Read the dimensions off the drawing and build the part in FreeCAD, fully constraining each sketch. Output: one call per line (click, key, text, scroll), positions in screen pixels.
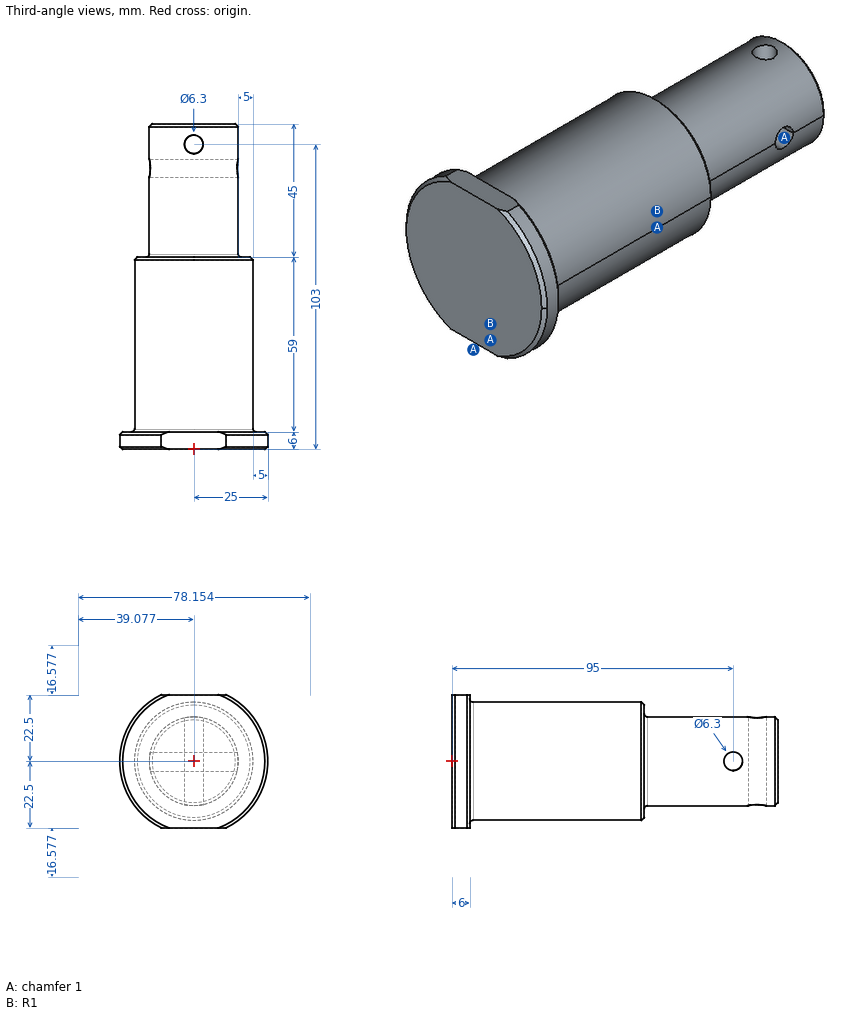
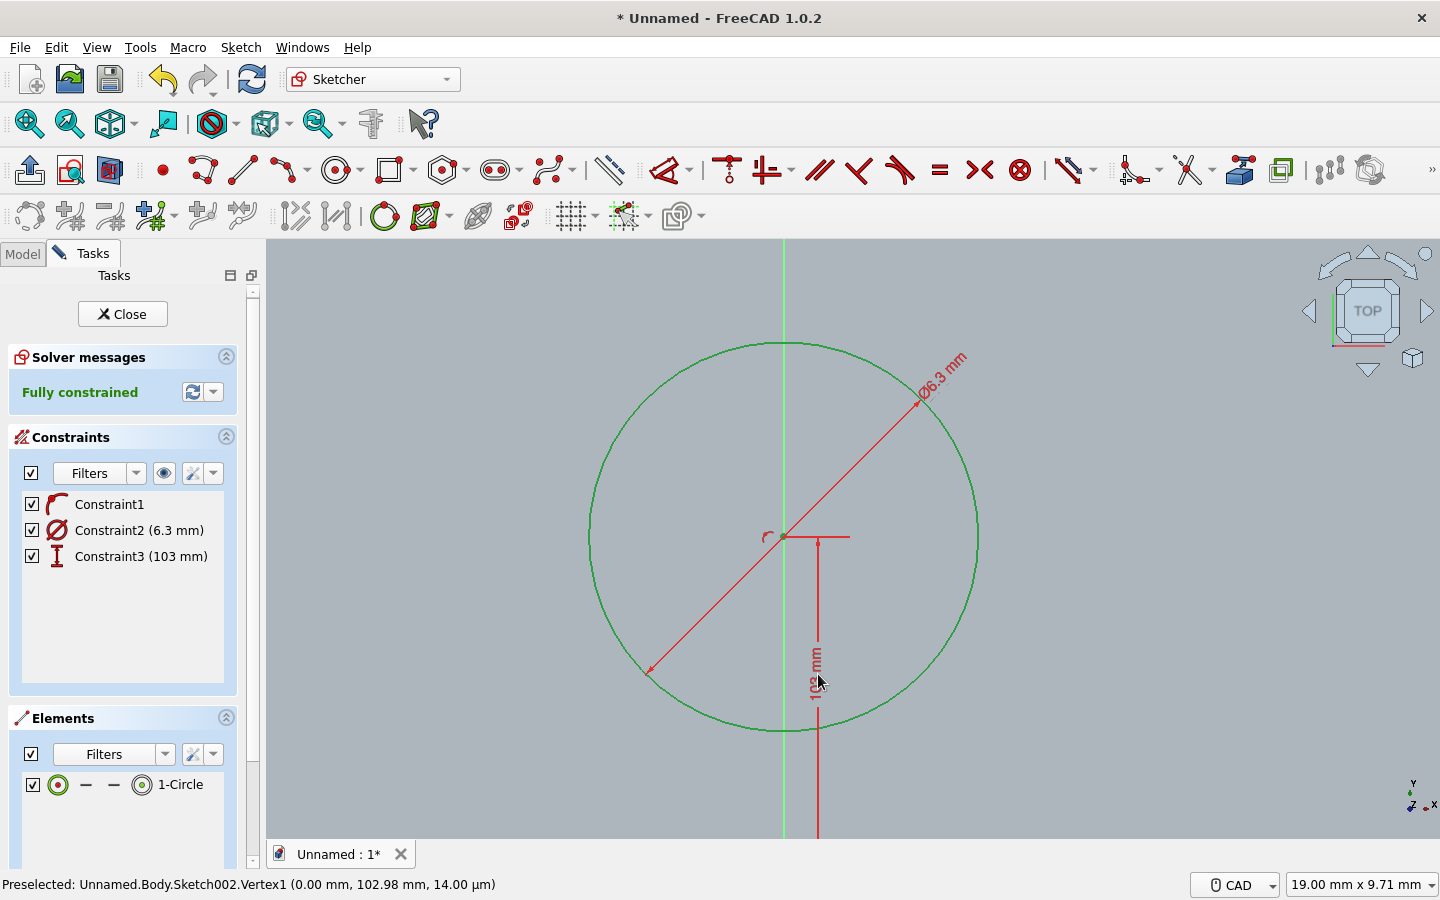
click(123, 314)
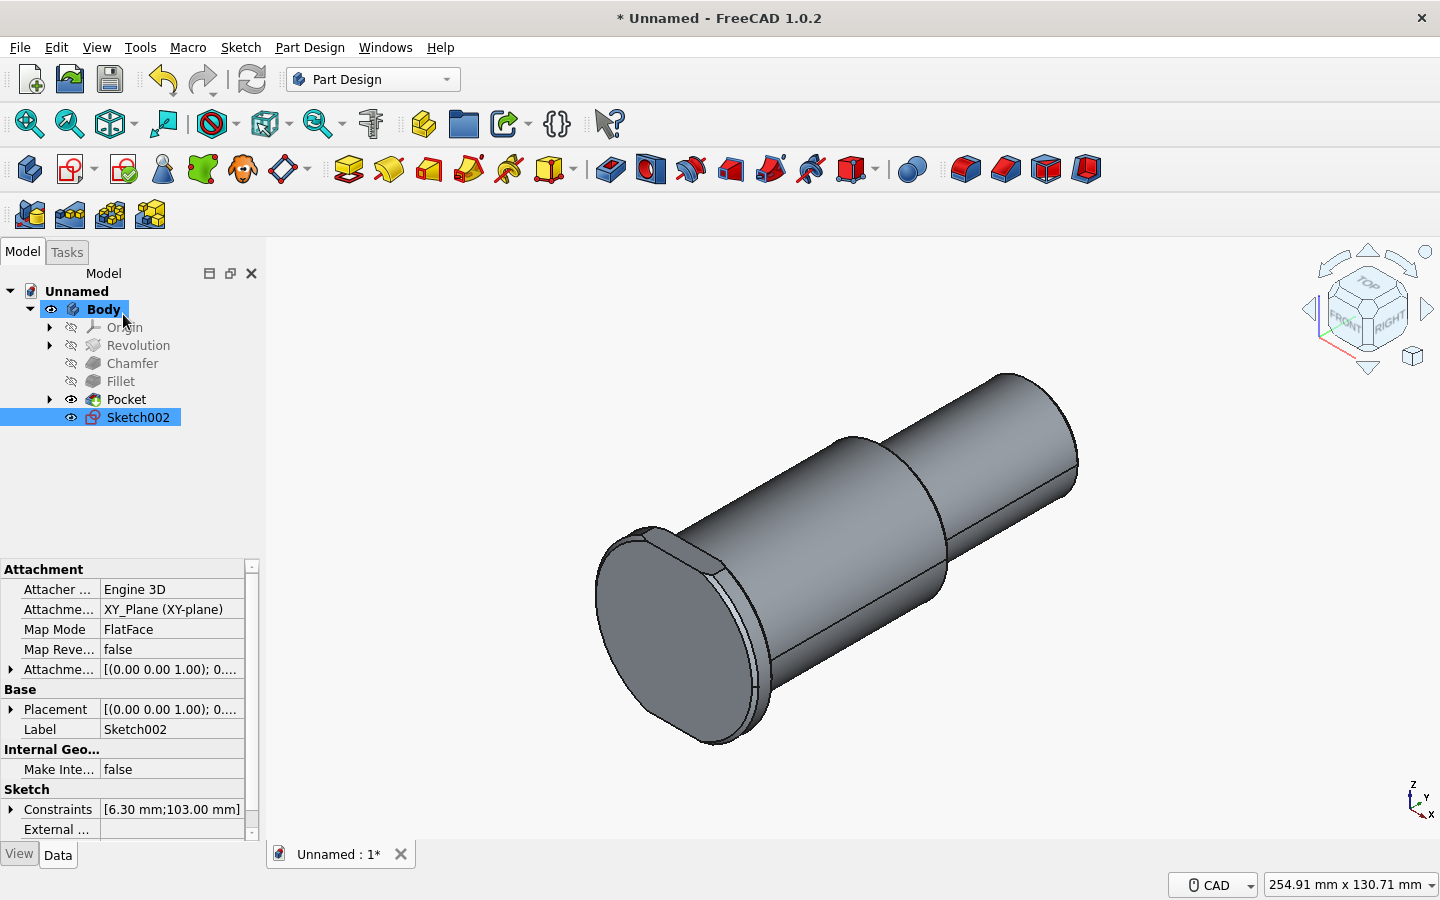
click(612, 170)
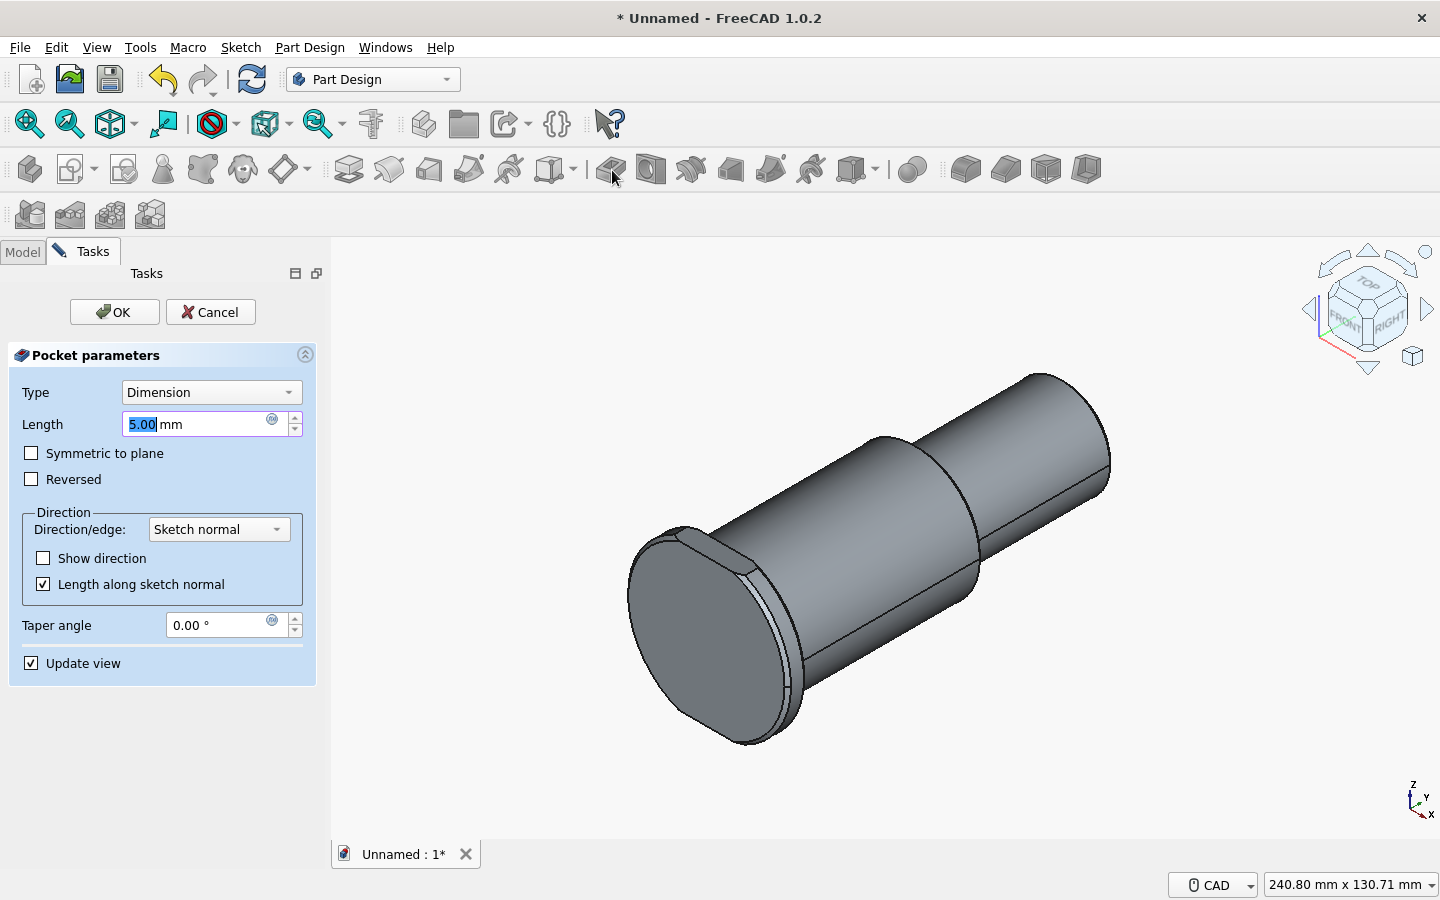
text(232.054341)
key(Tab)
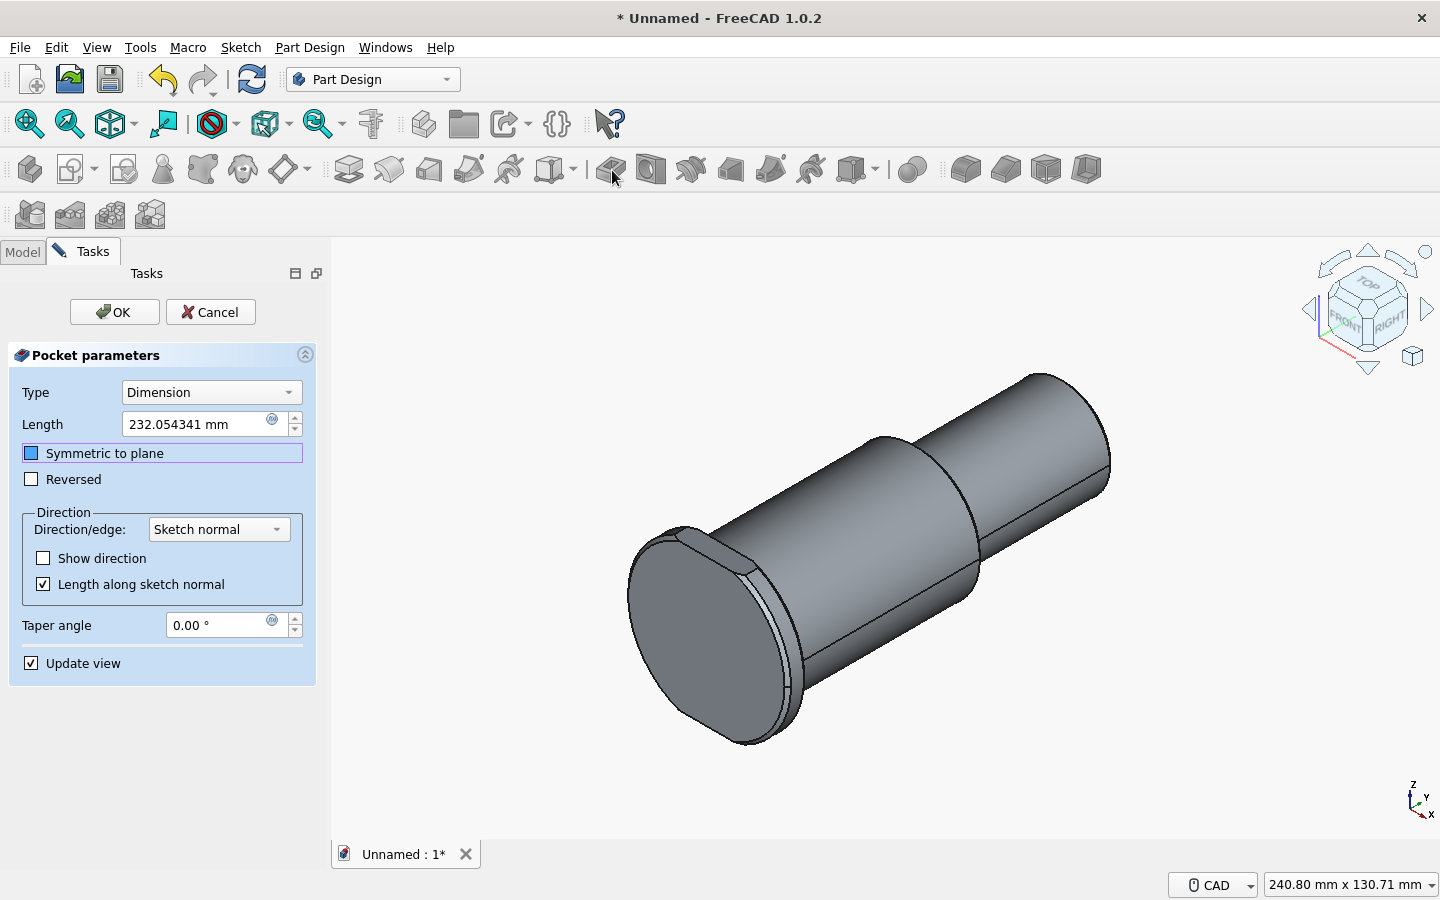
click(30, 453)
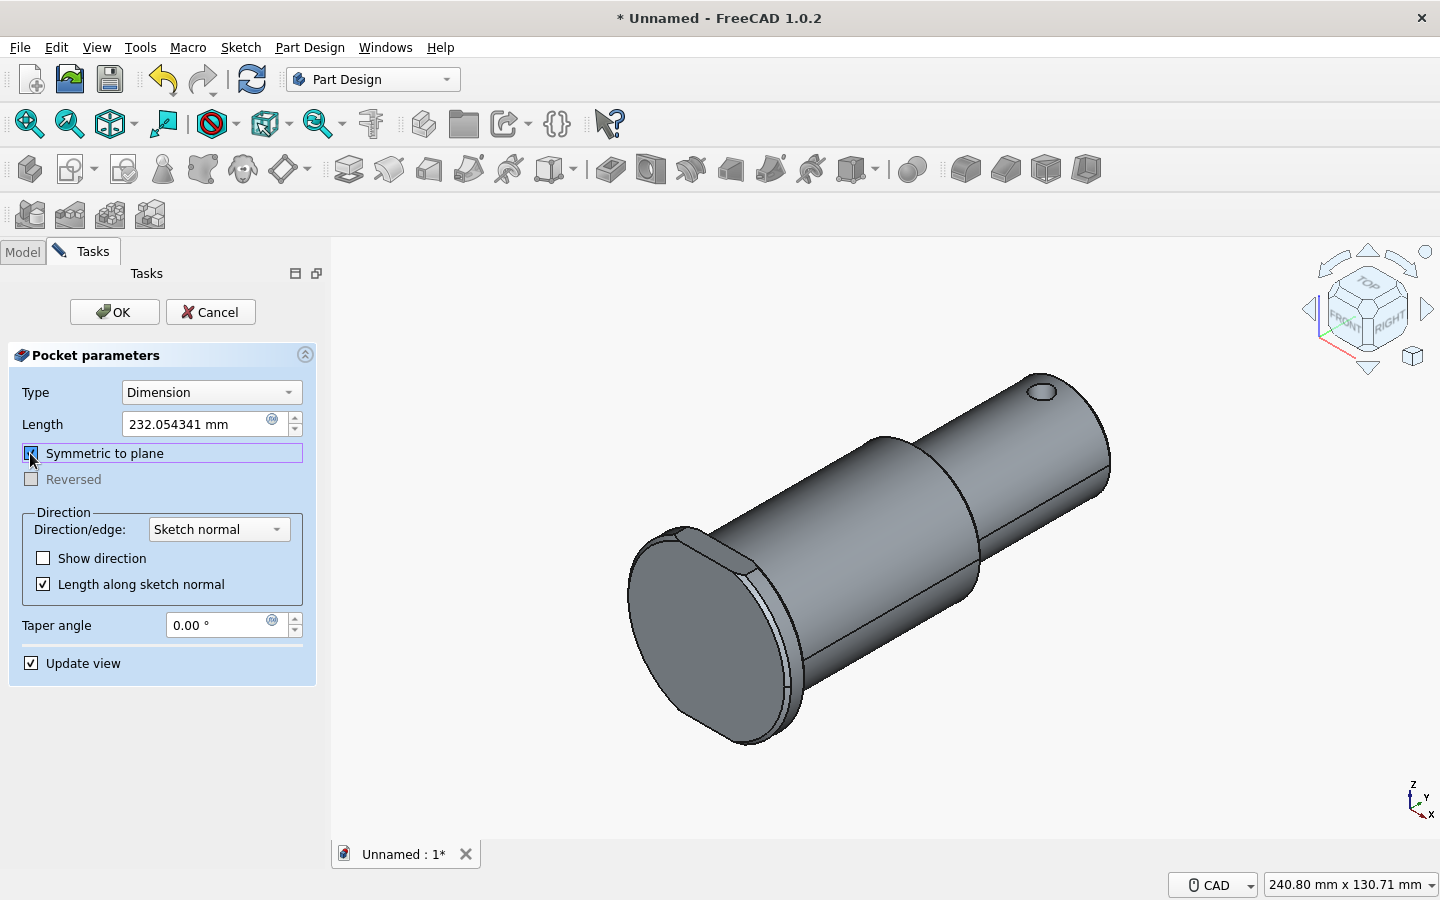
click(115, 312)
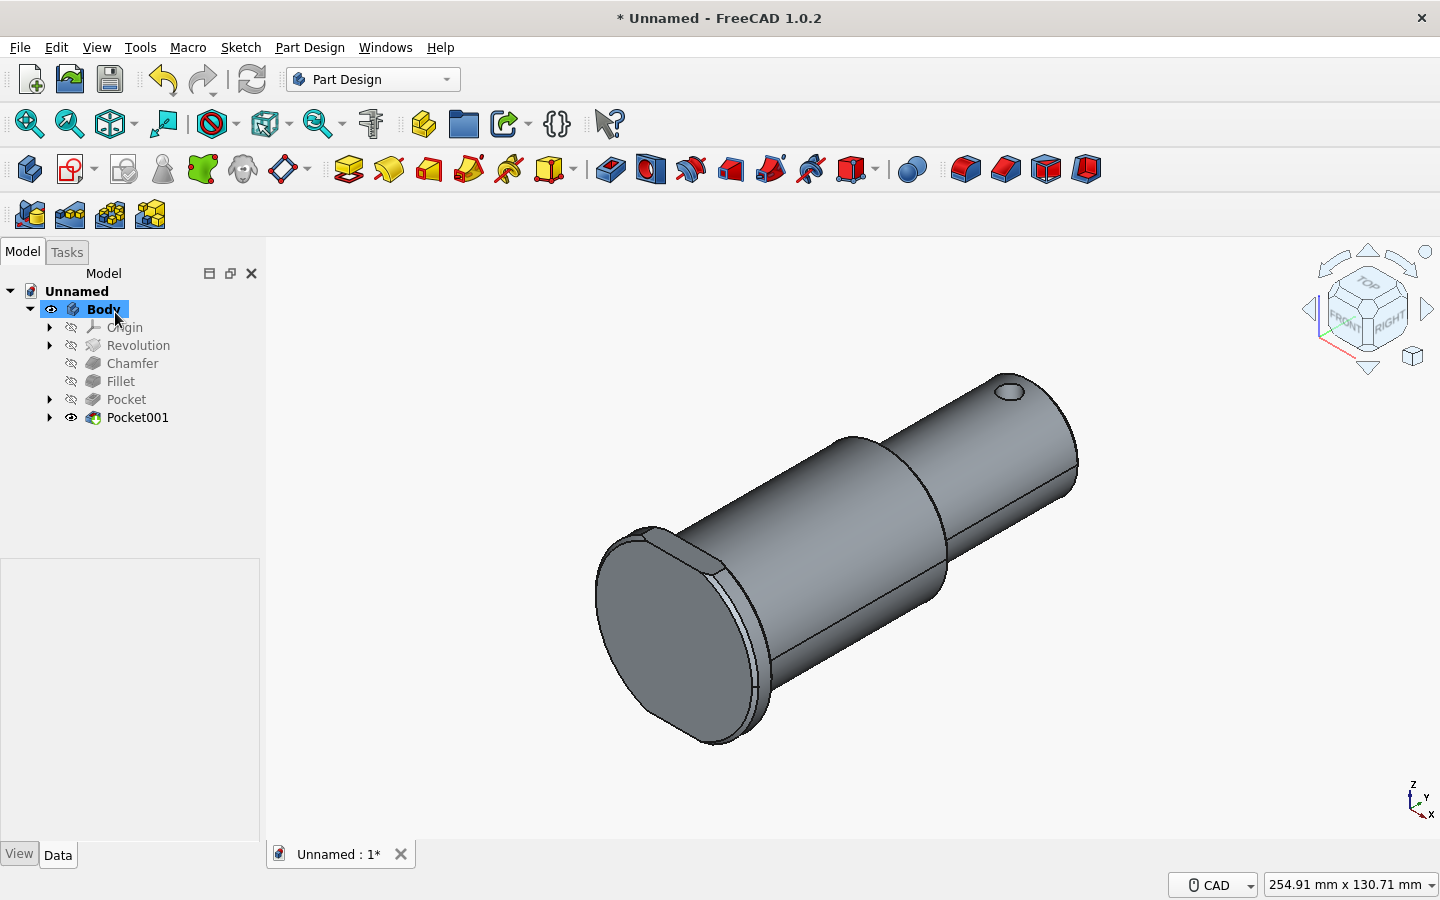
click(70, 170)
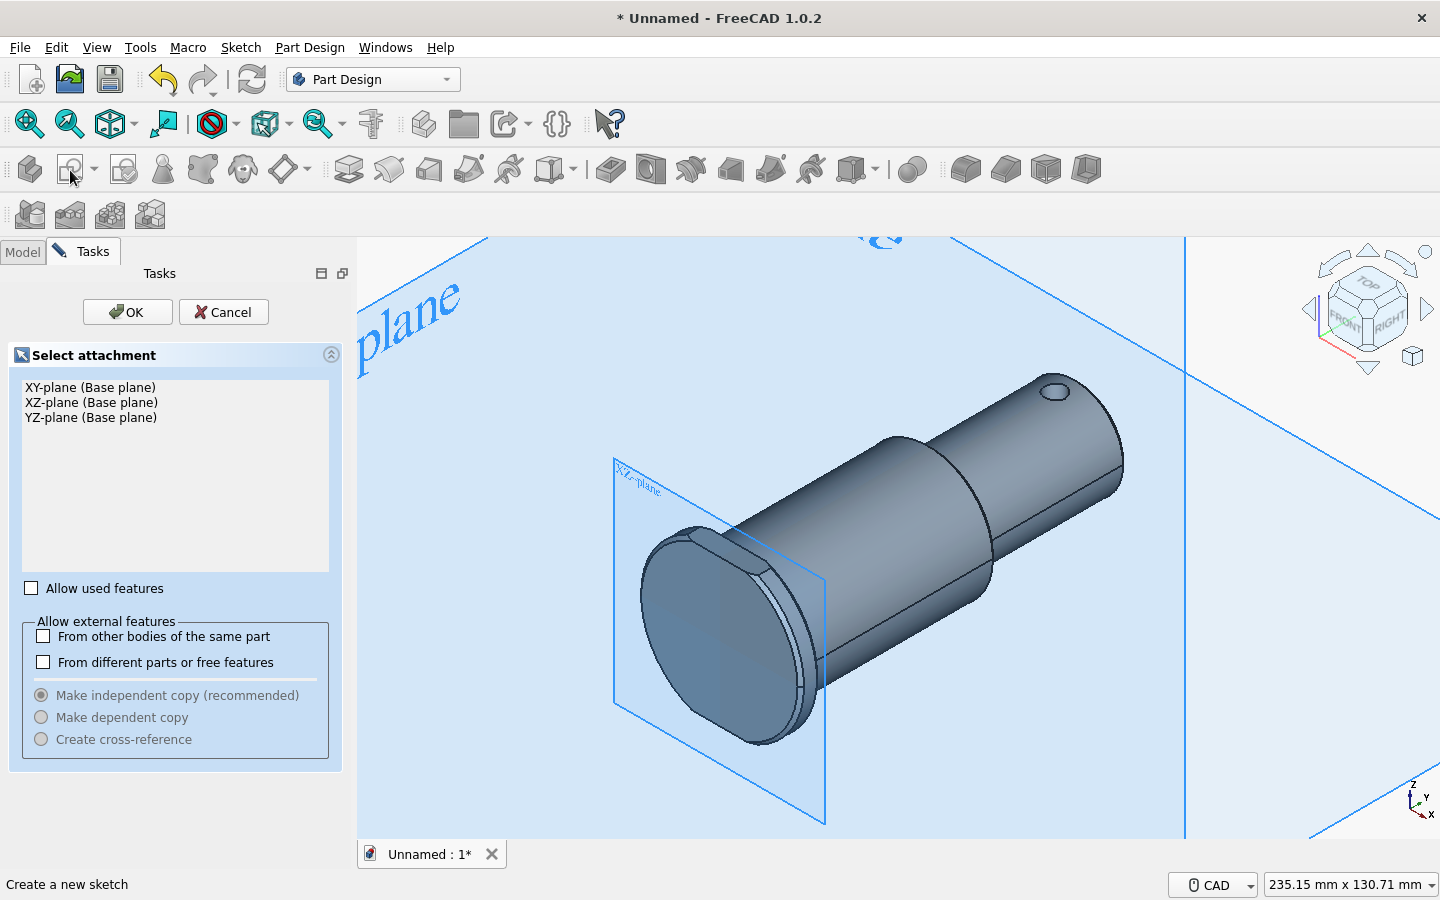
click(82, 418)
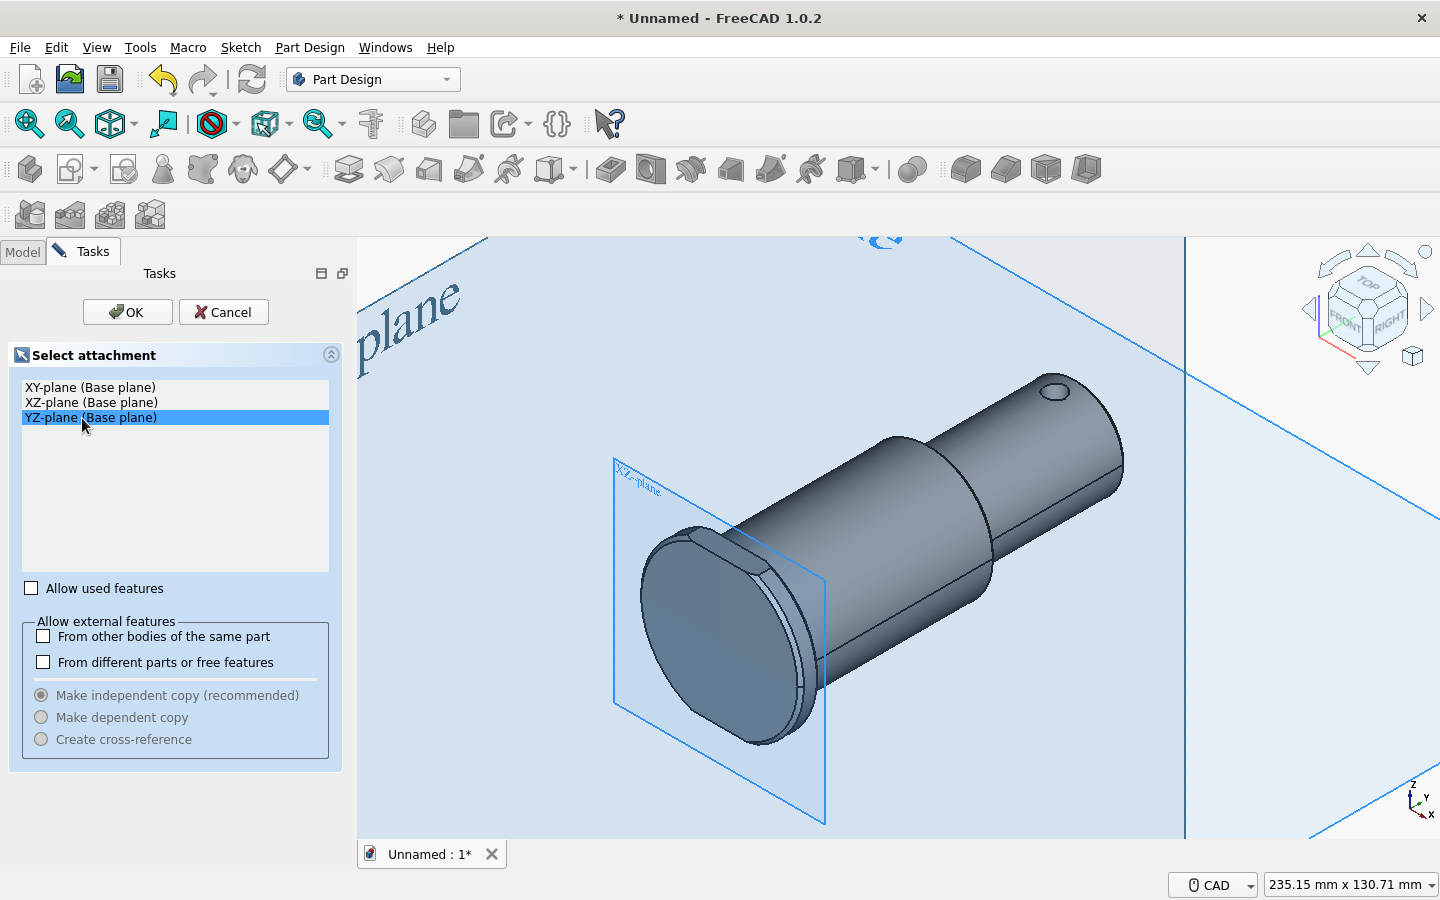
click(128, 312)